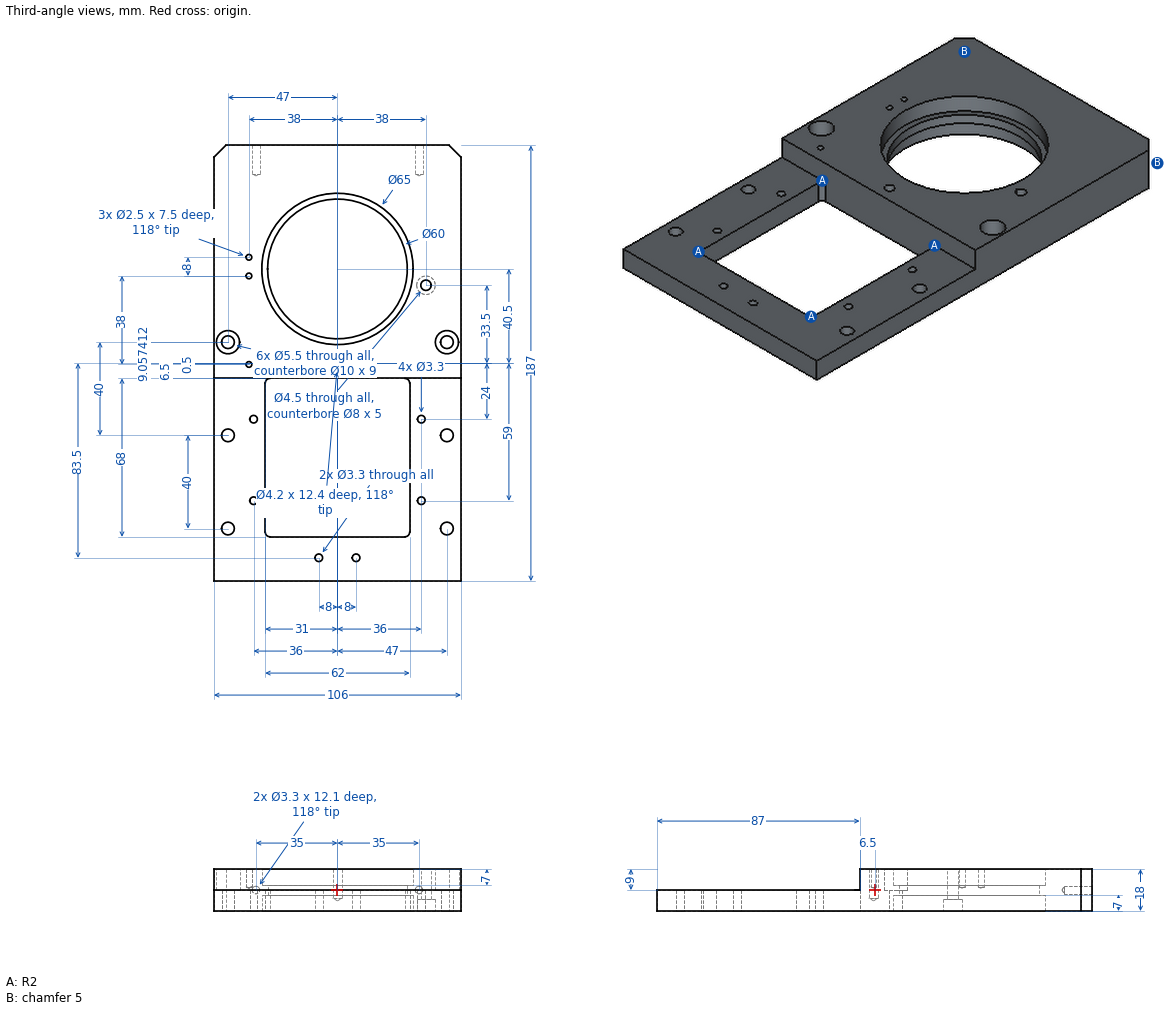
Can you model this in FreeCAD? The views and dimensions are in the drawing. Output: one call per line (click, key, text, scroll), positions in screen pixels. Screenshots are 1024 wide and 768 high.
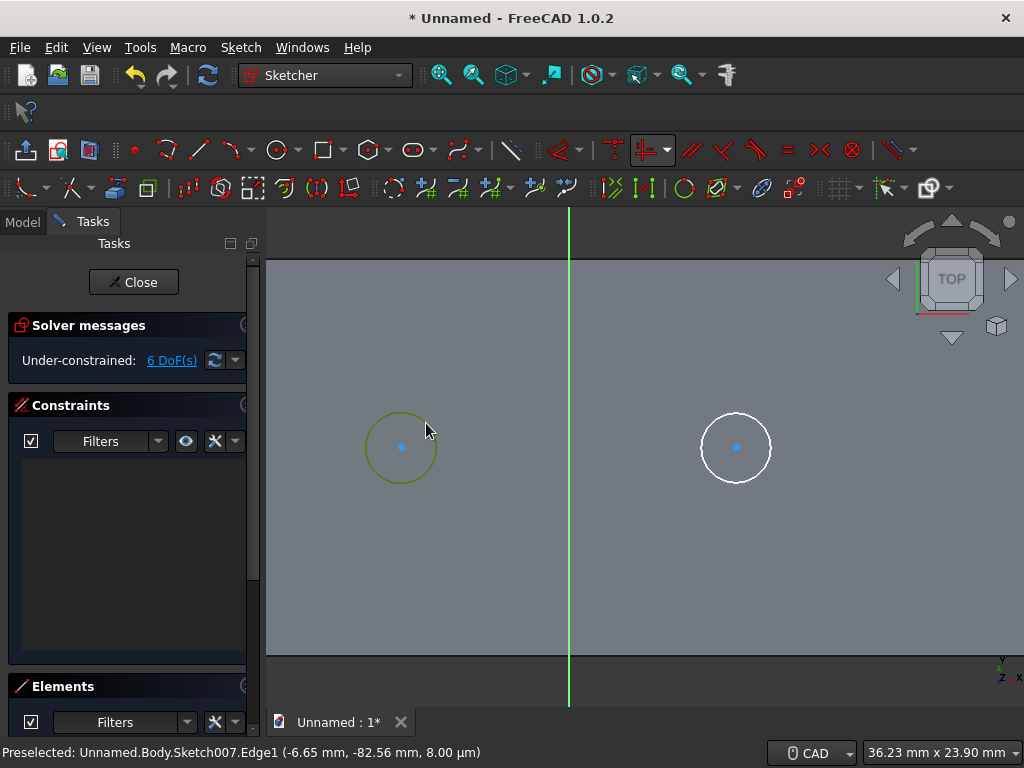
click(760, 423)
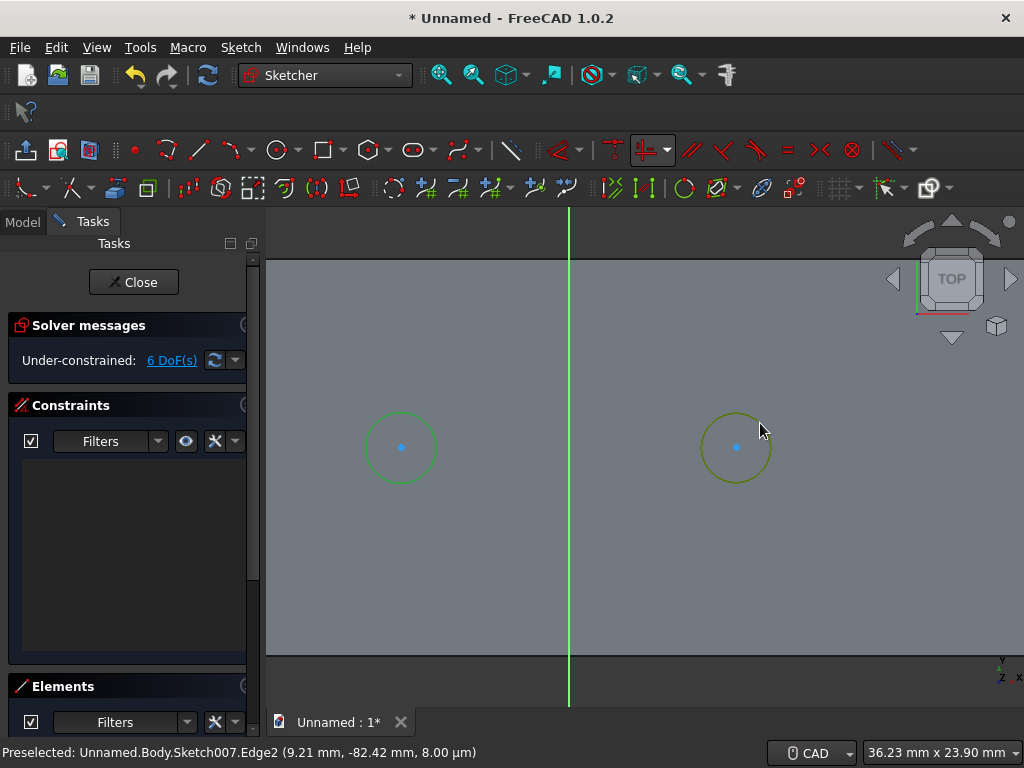
click(788, 150)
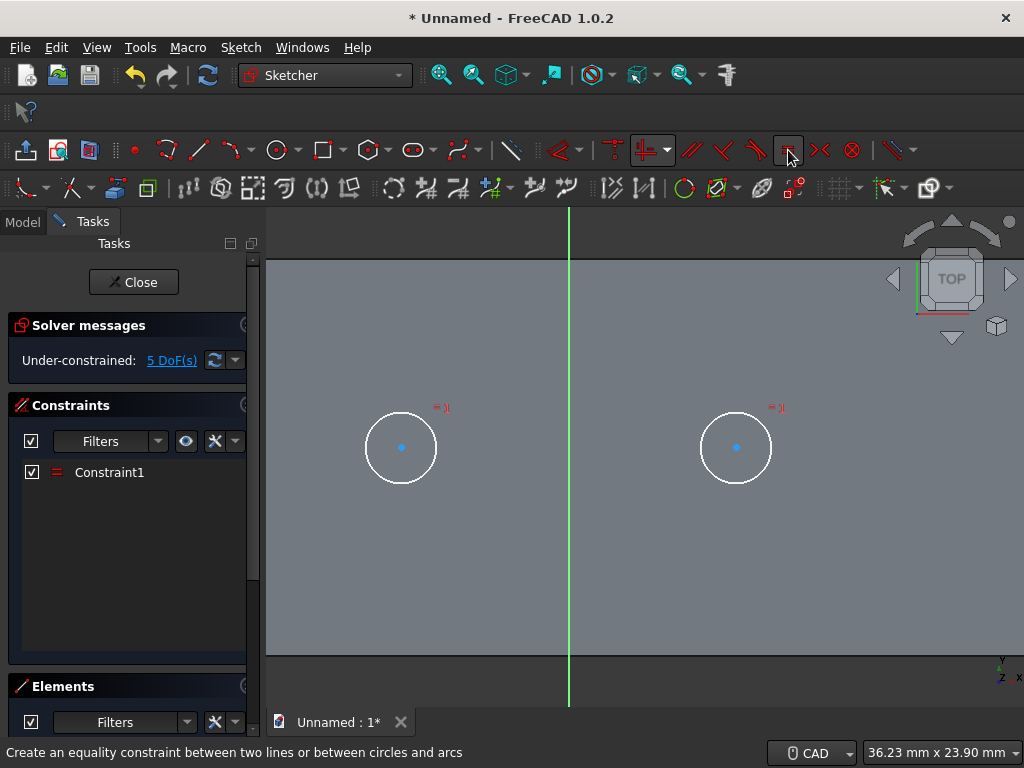
click(401, 448)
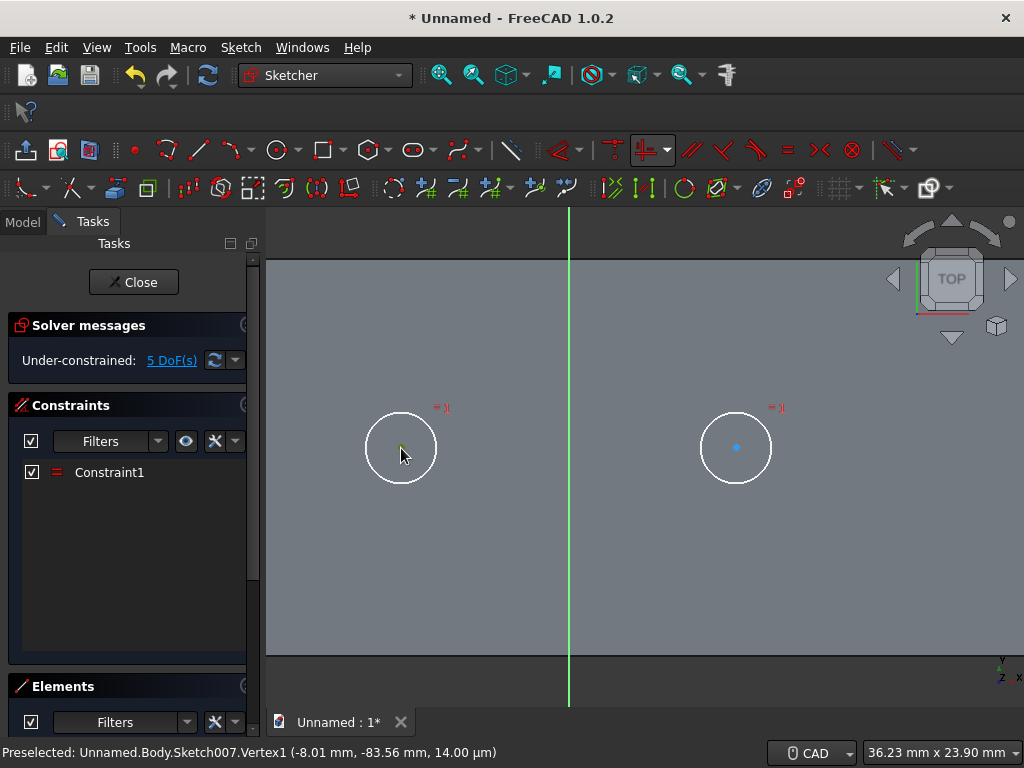
click(736, 448)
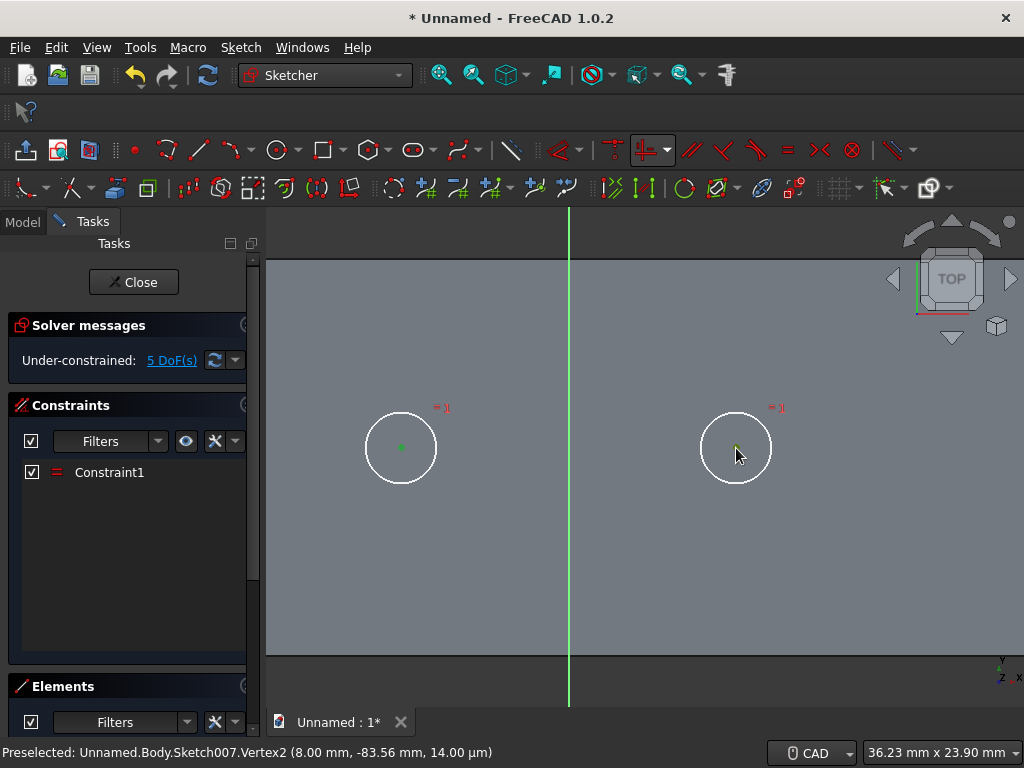
click(670, 150)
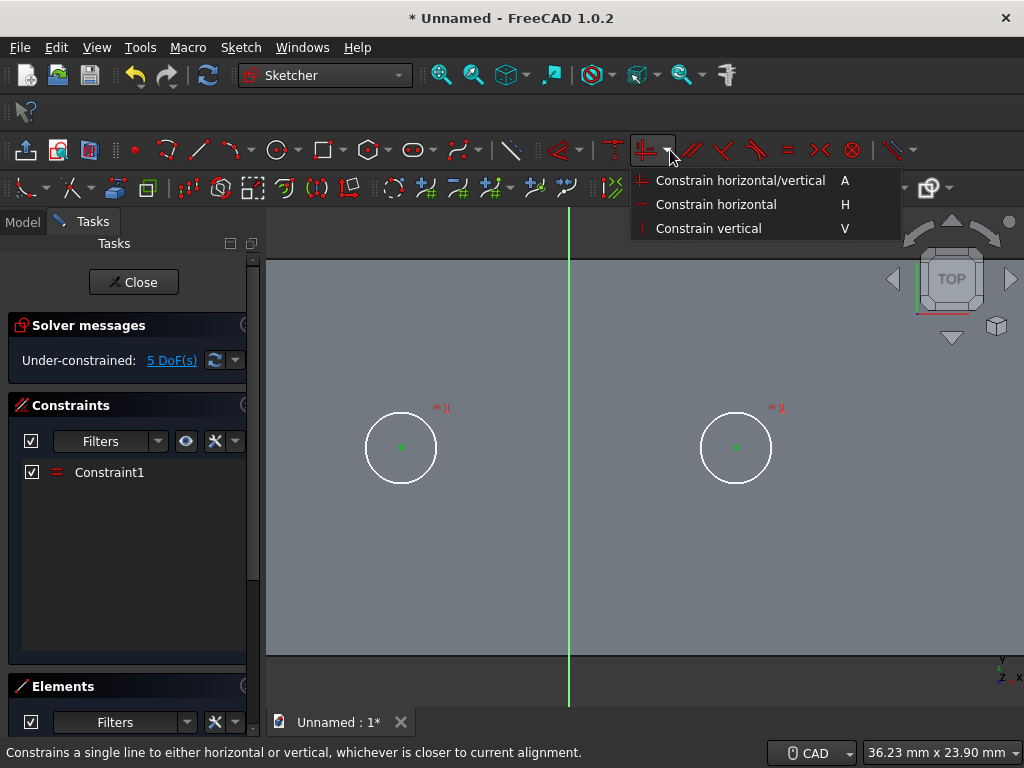
click(766, 204)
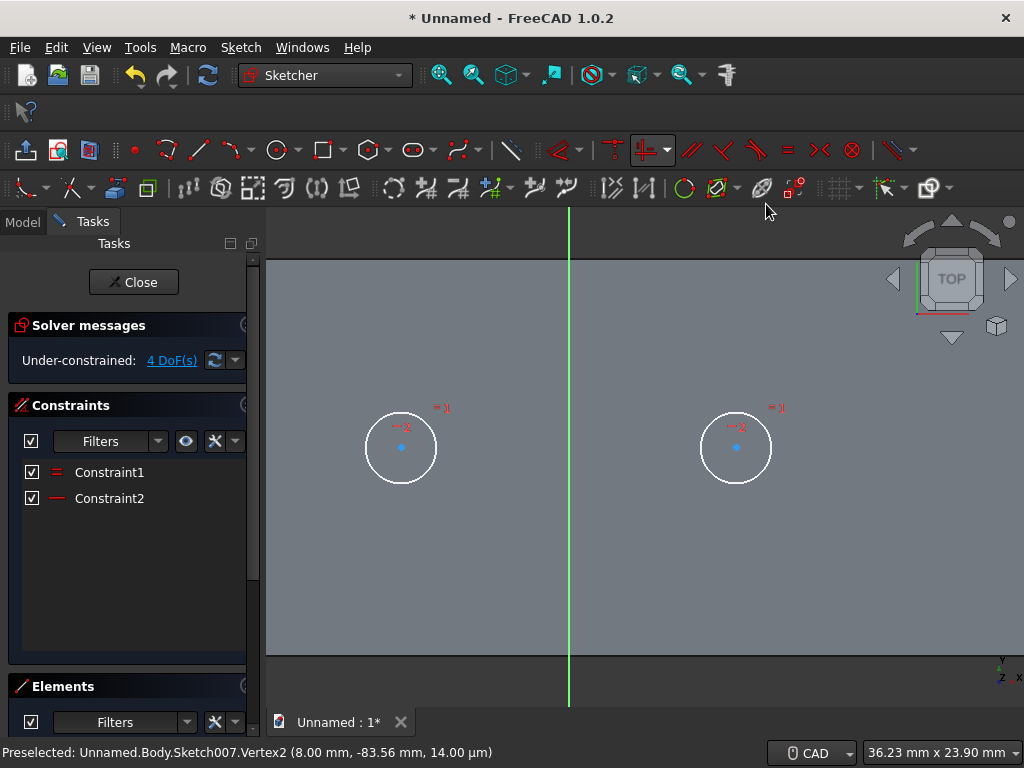
click(558, 150)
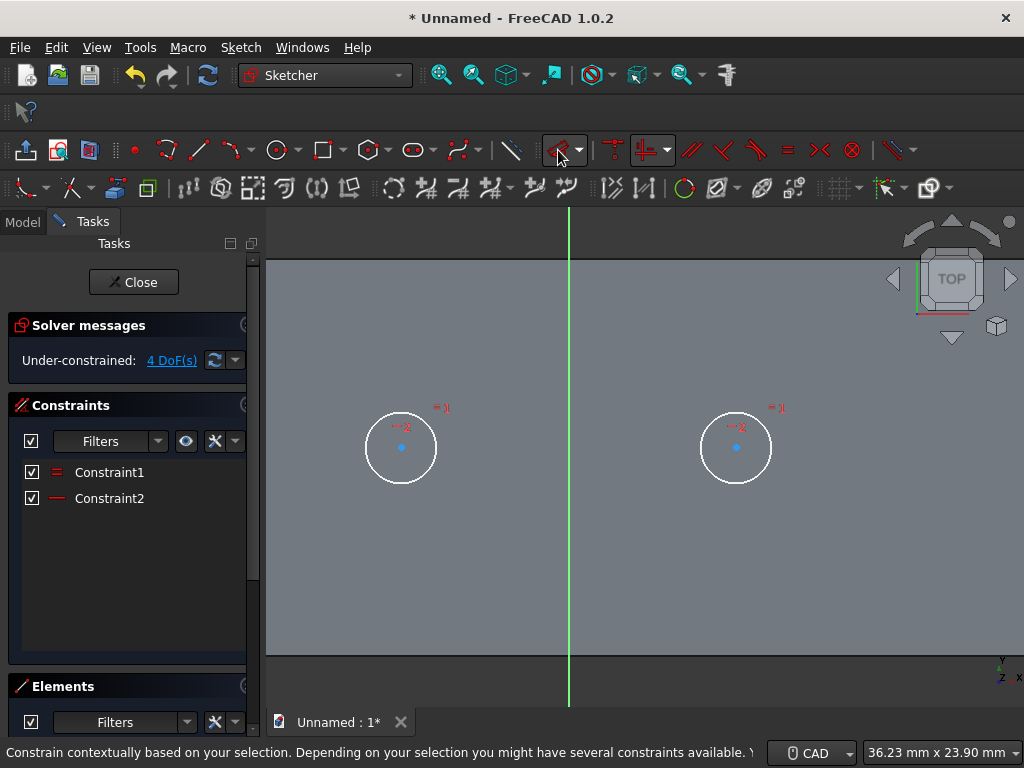
click(426, 423)
click(449, 400)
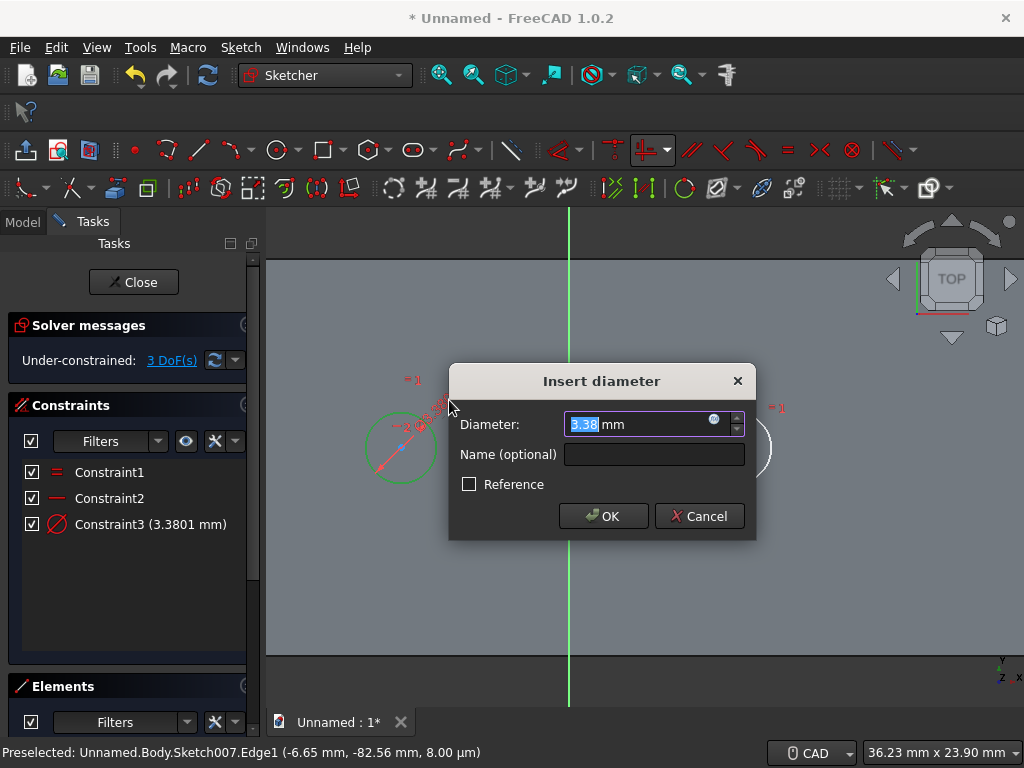
text(3.3)
key(Return)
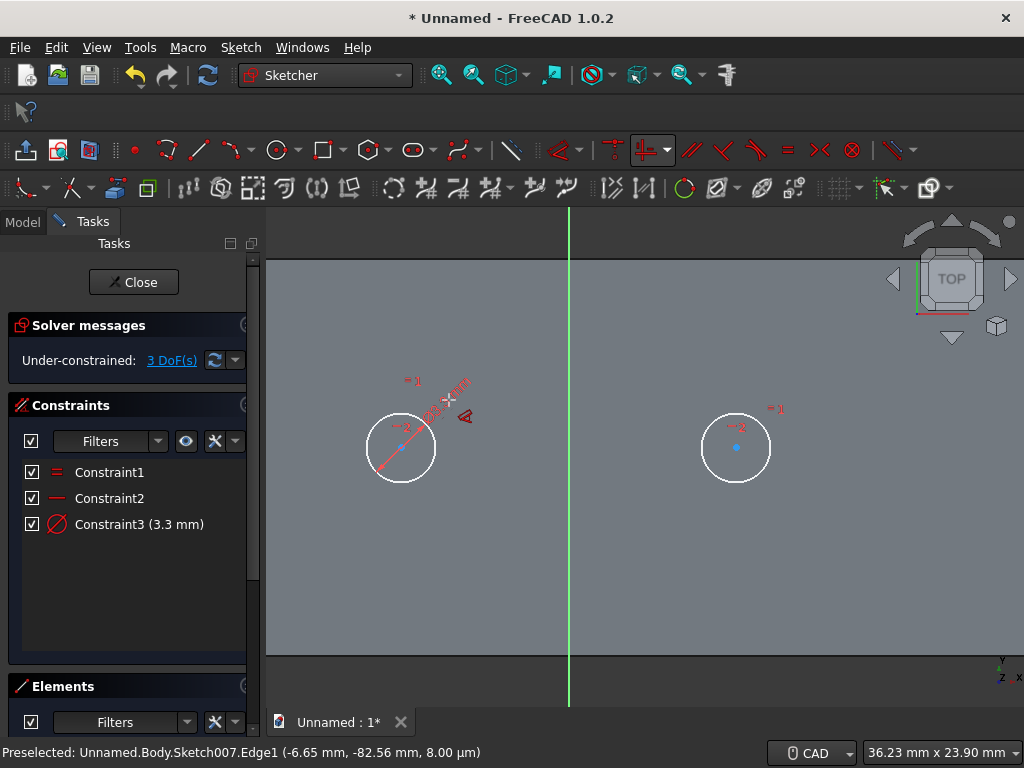
click(401, 448)
click(485, 482)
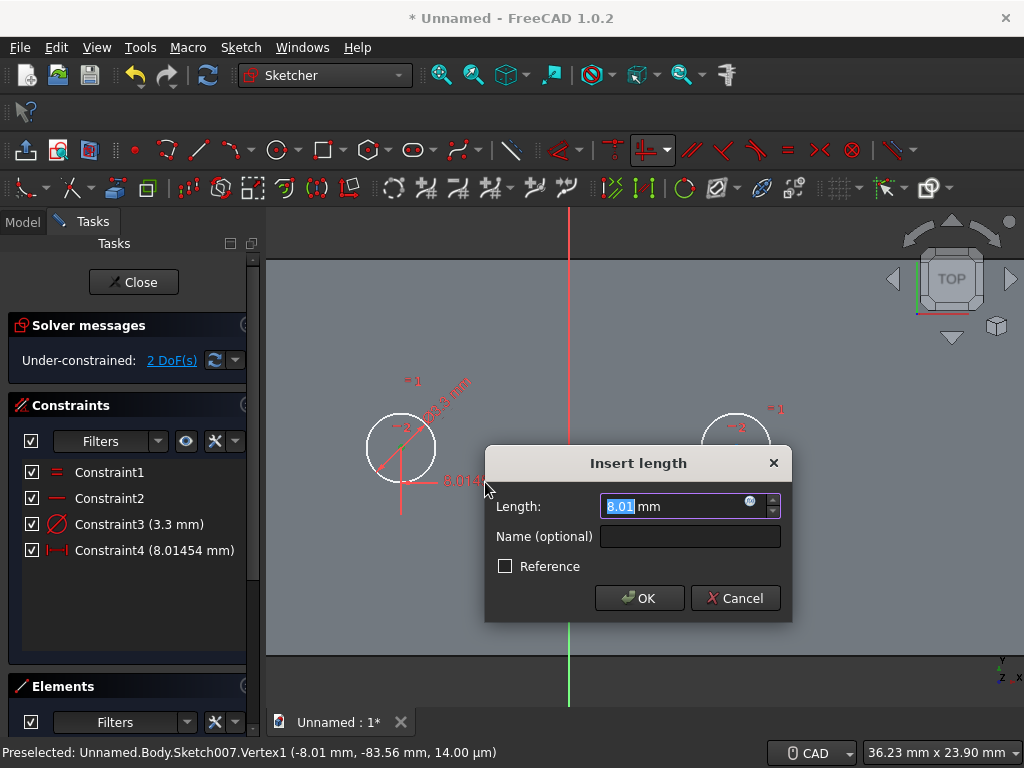
text(8)
key(Return)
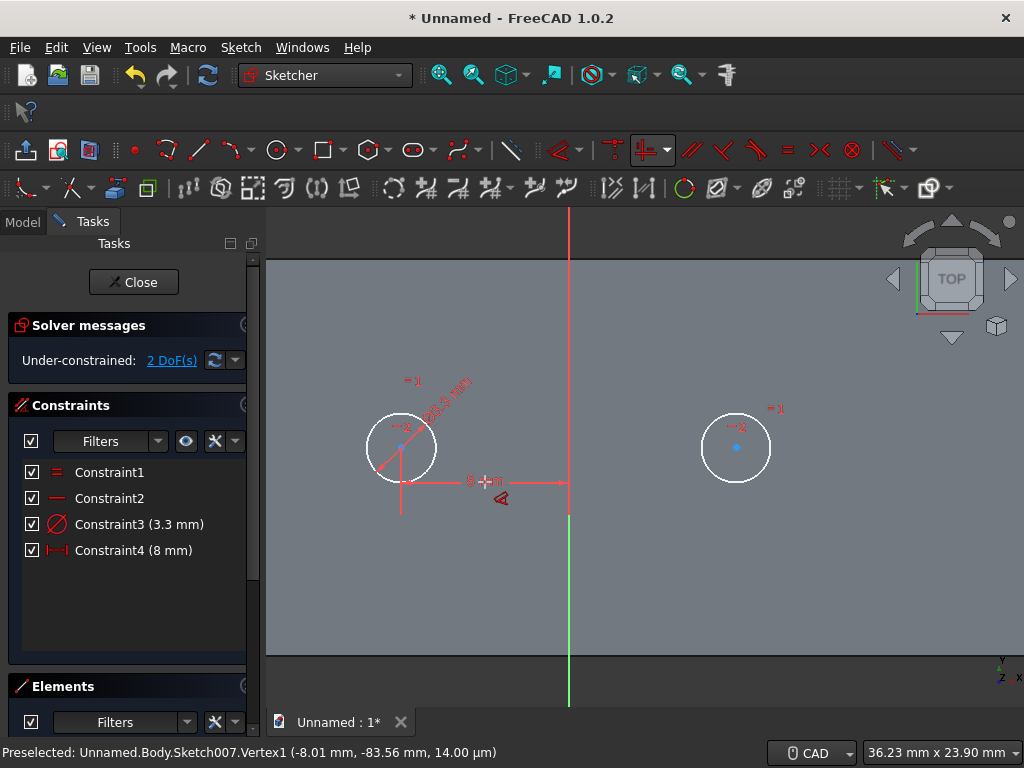
click(736, 448)
click(652, 482)